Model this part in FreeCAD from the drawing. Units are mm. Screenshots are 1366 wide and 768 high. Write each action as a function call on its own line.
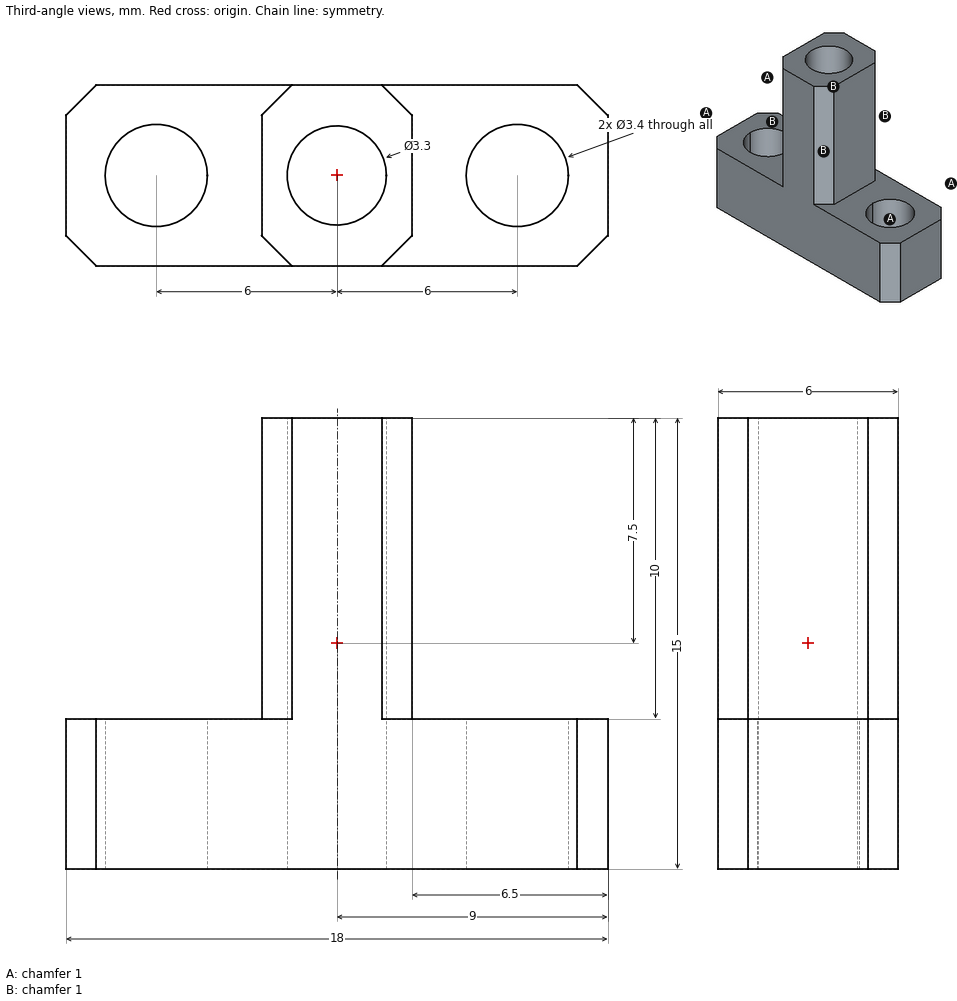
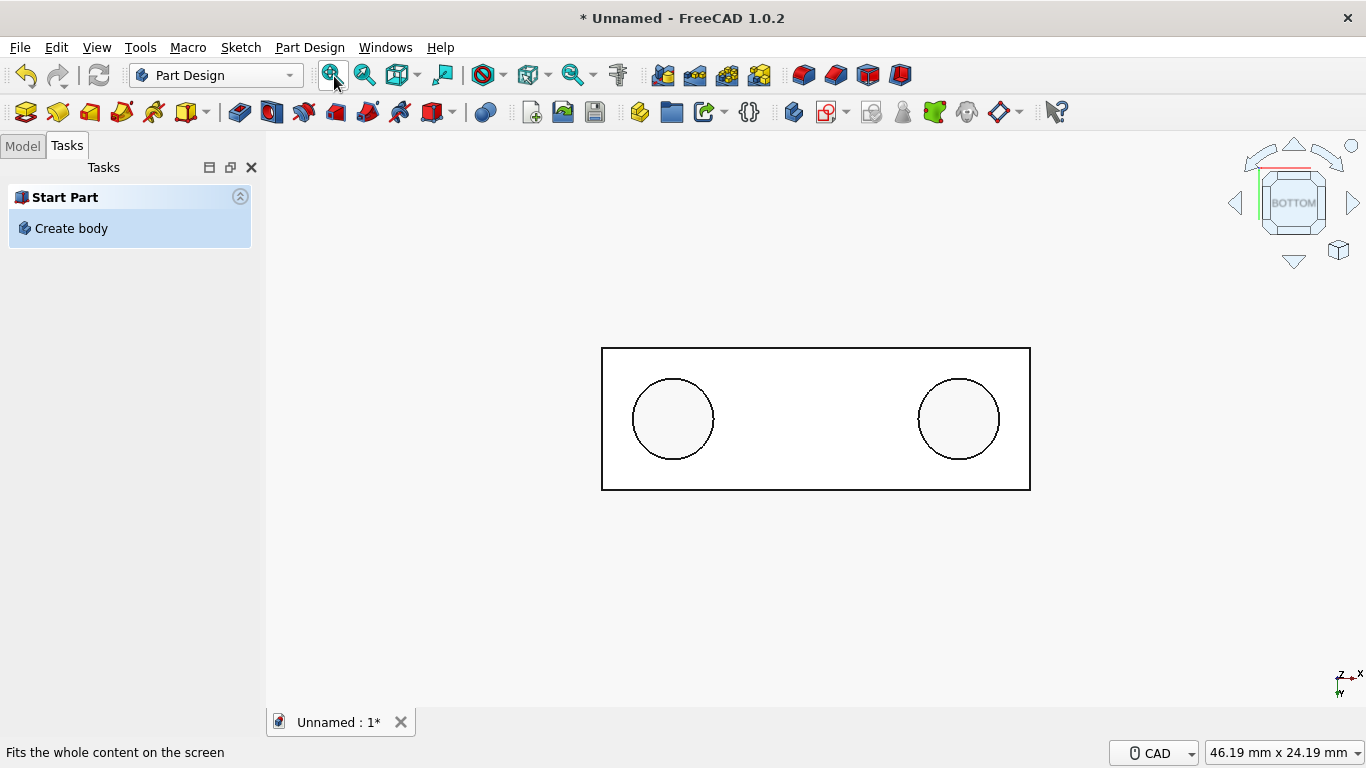
key(0)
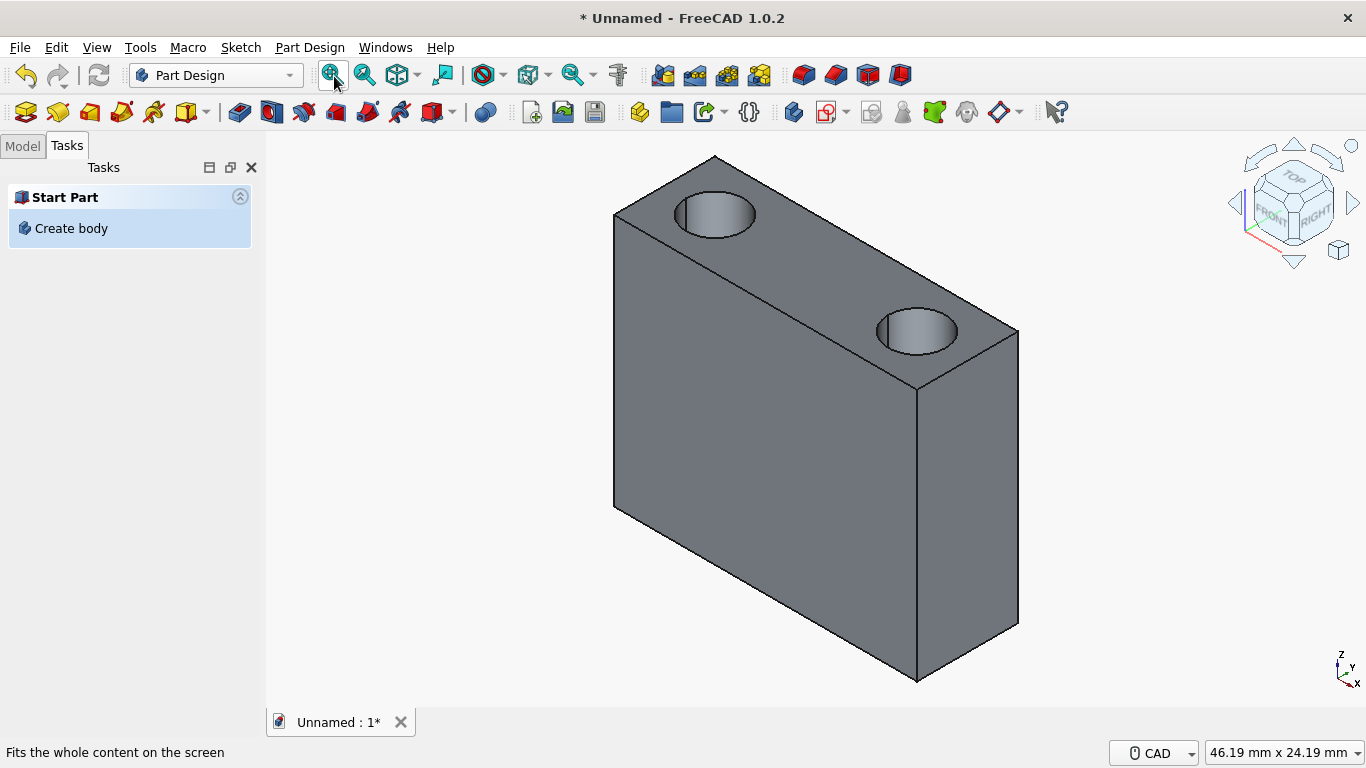
click(917, 535)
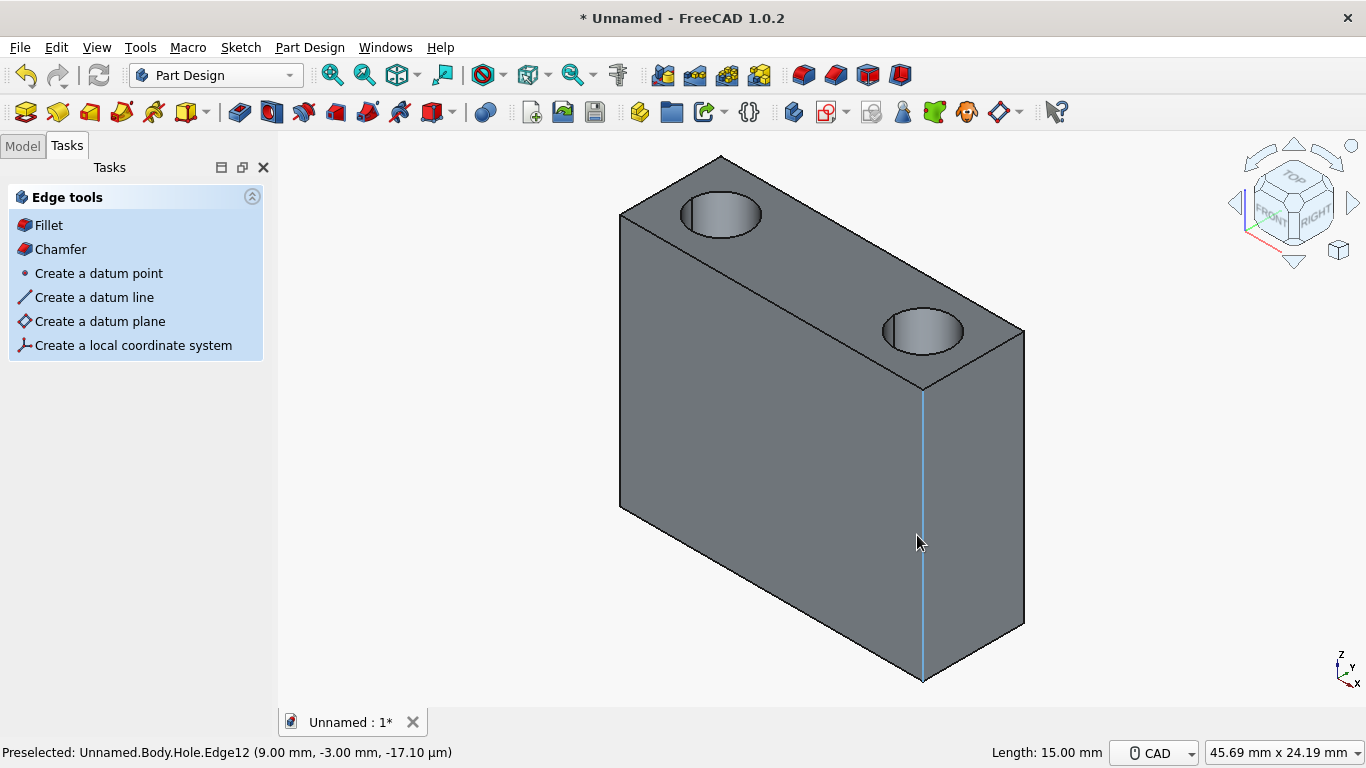
key(2)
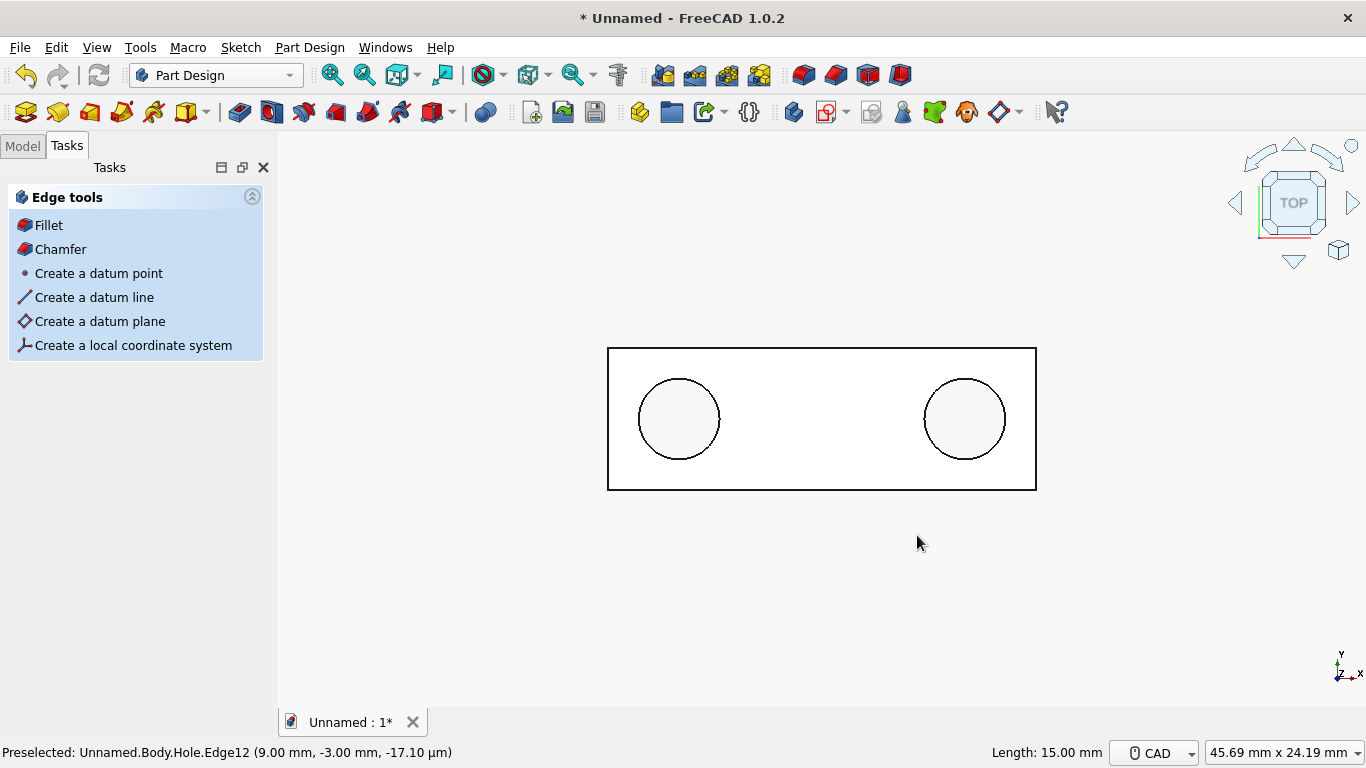
click(334, 76)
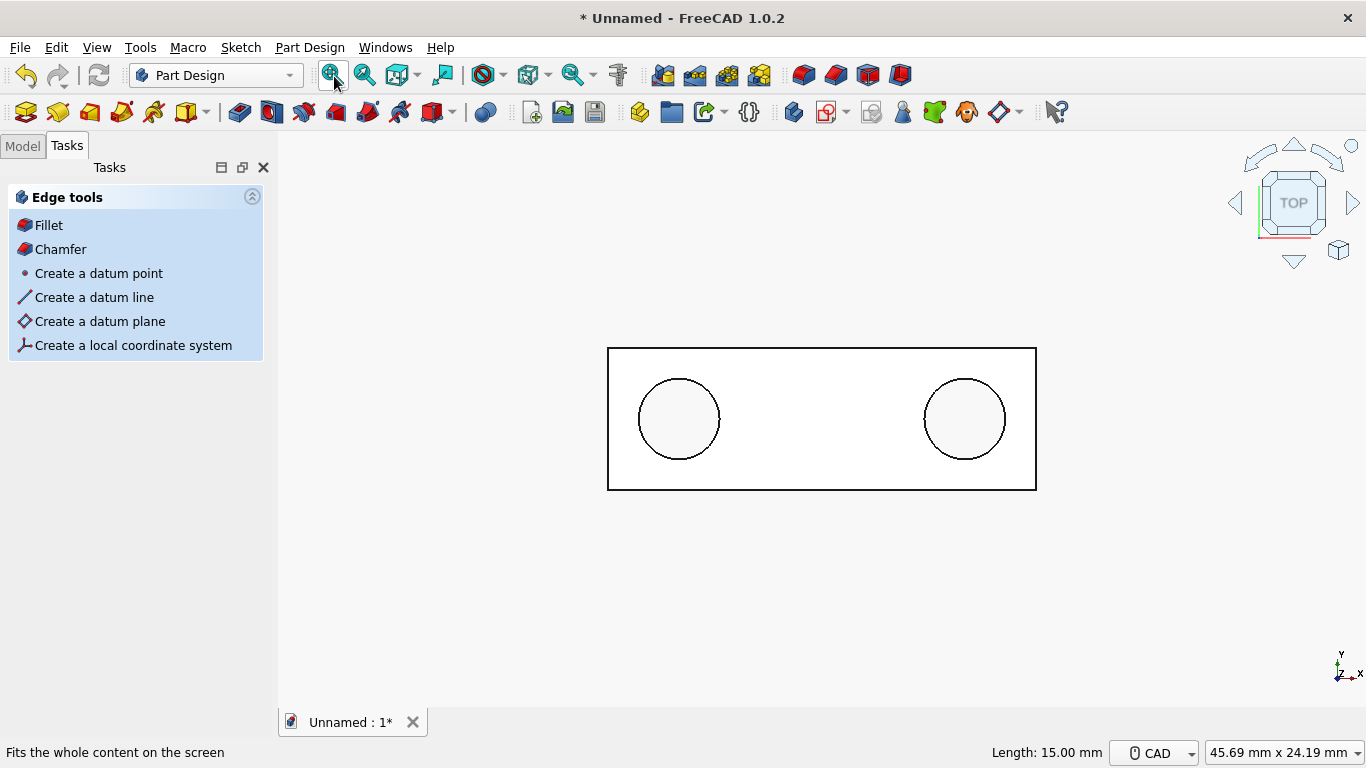
key(1)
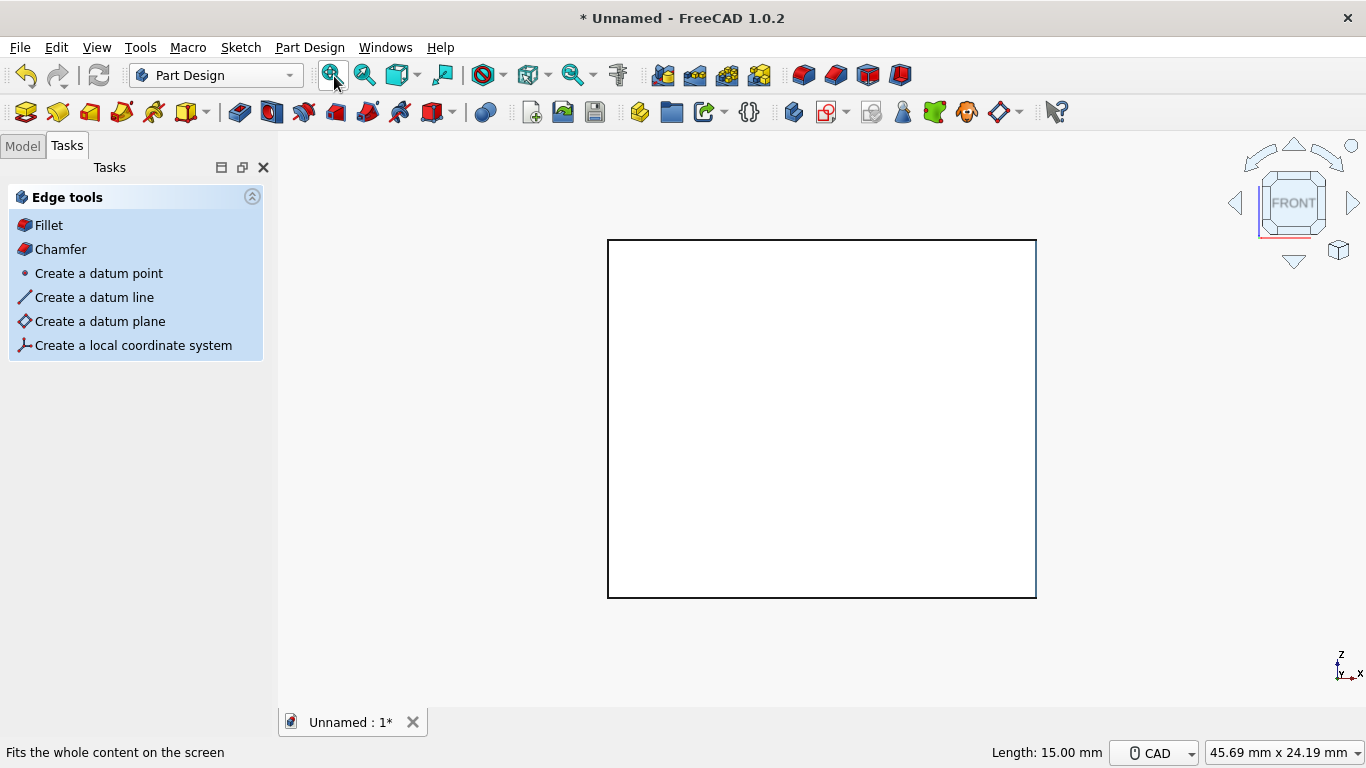
click(608, 418, ctrl)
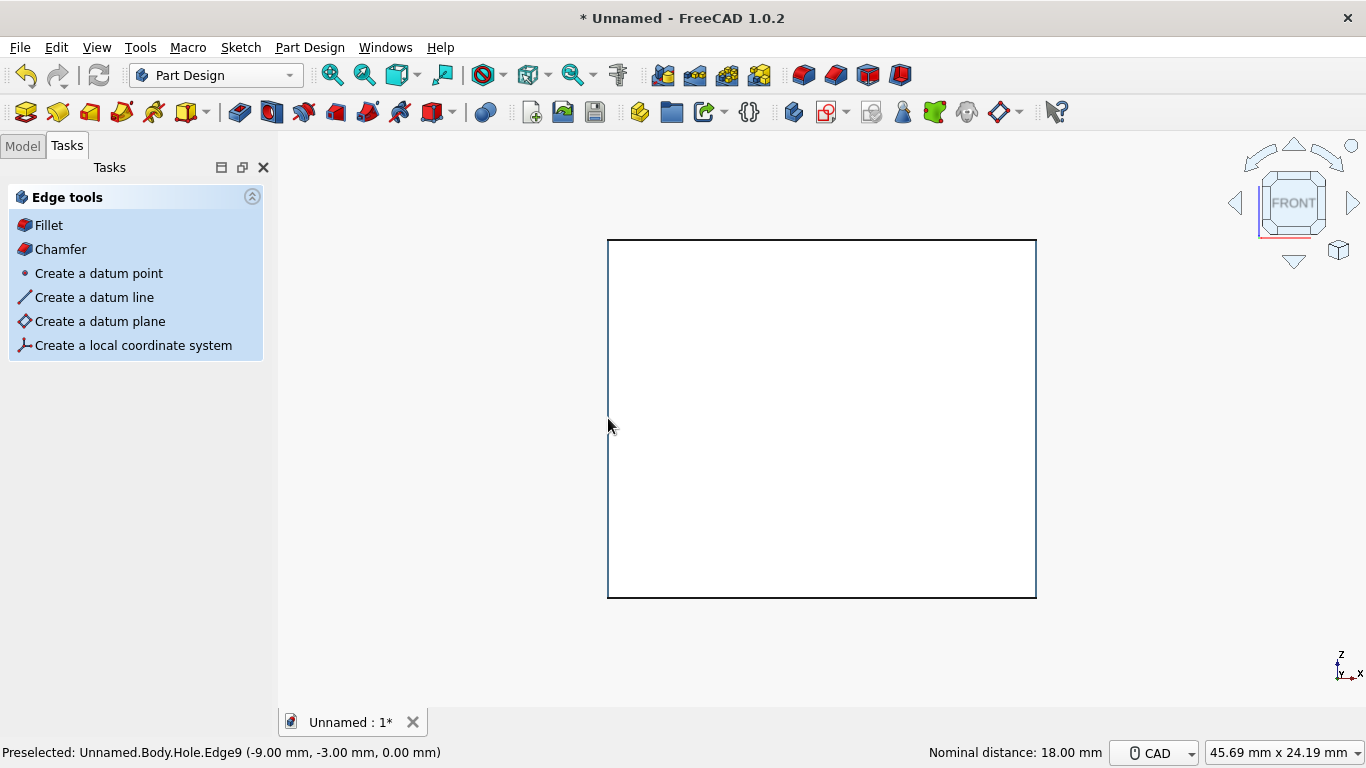
key(3)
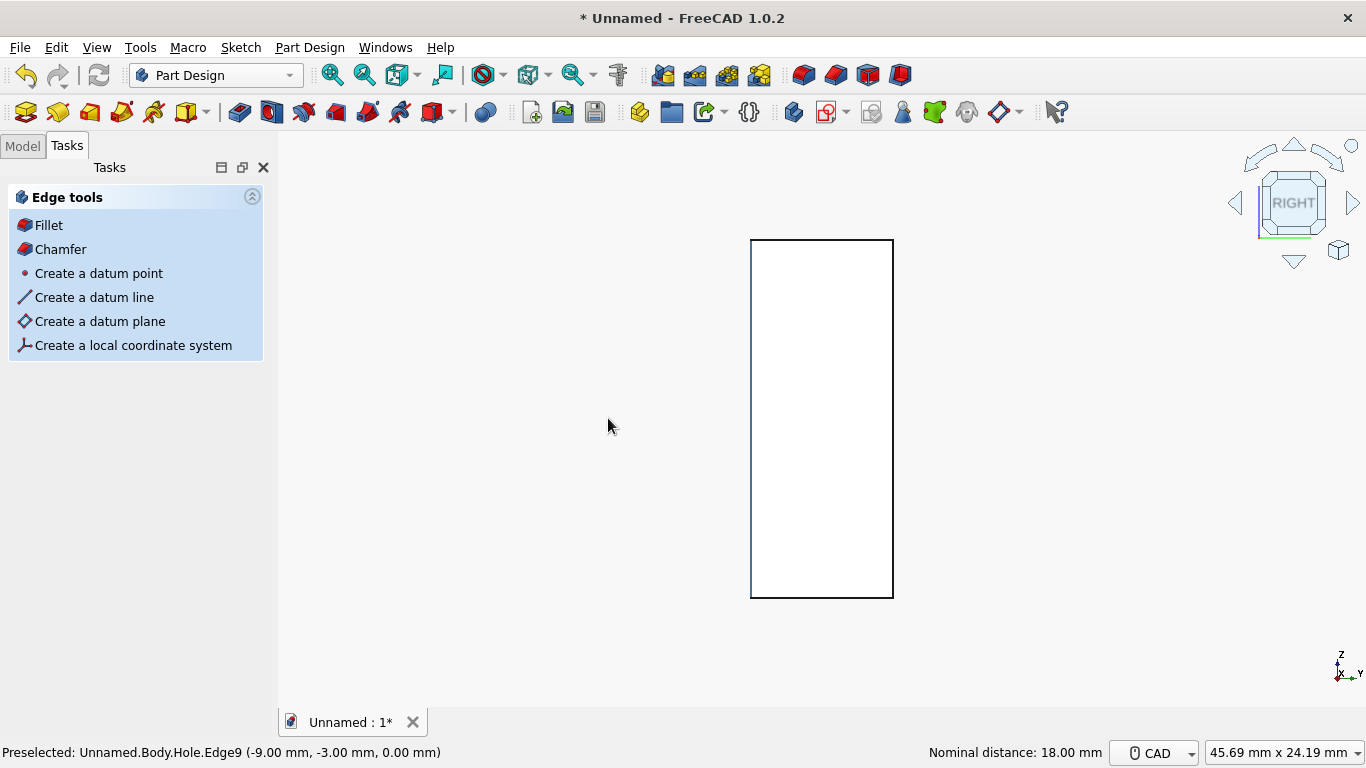
click(893, 418, ctrl)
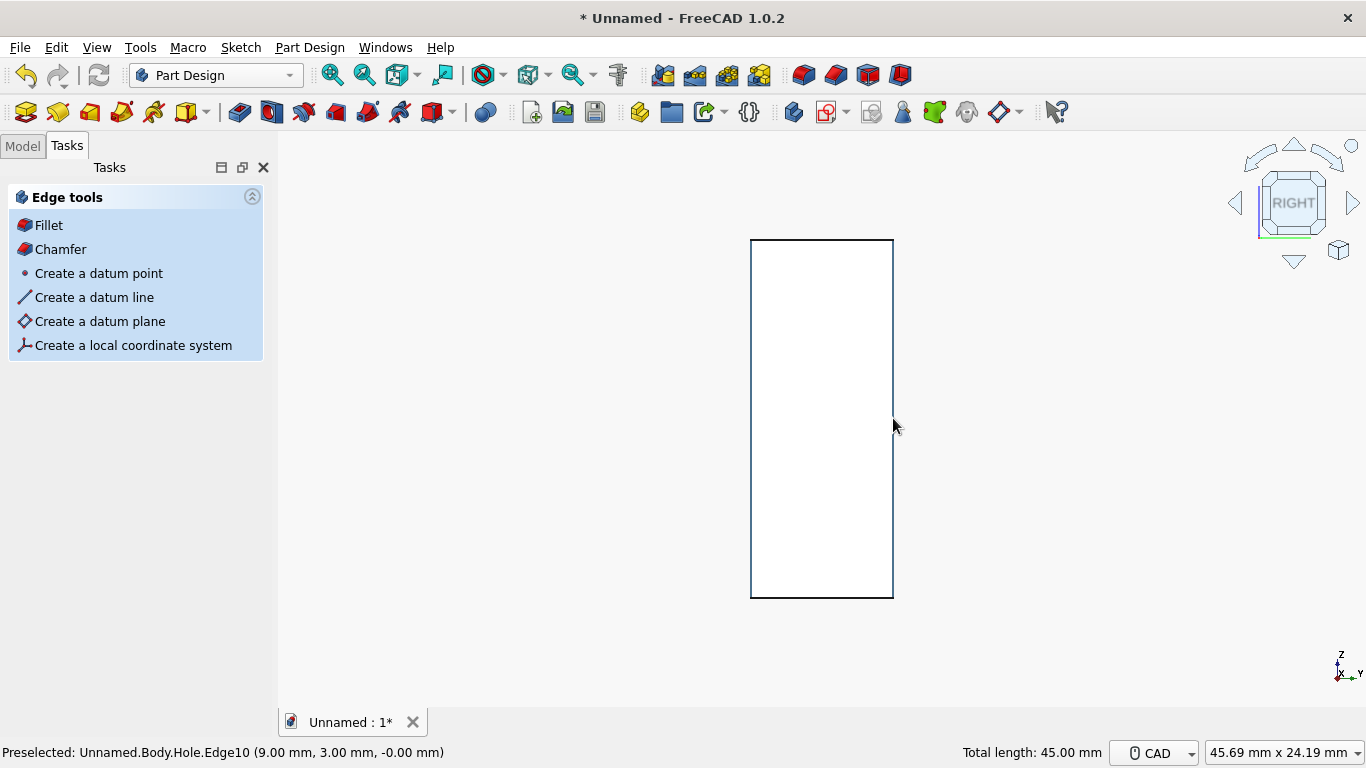
key(5)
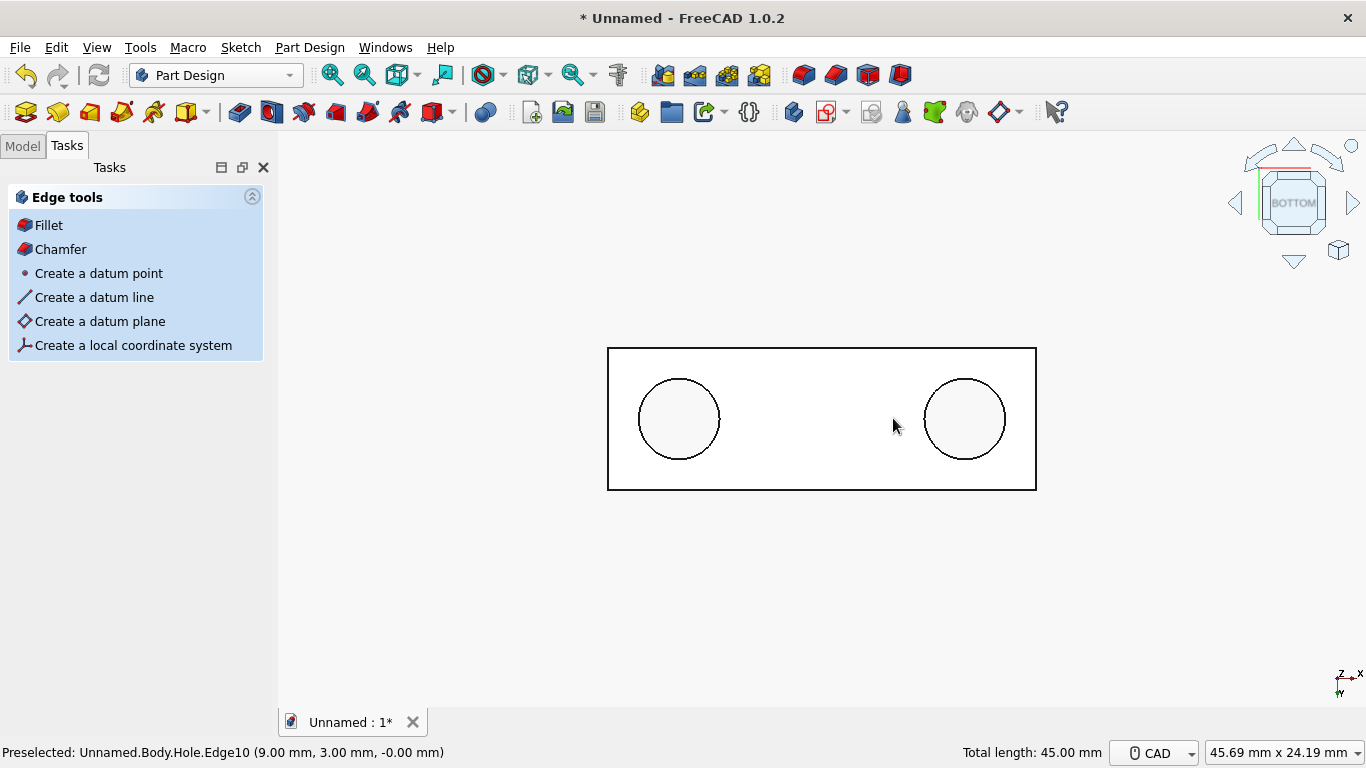
click(334, 76)